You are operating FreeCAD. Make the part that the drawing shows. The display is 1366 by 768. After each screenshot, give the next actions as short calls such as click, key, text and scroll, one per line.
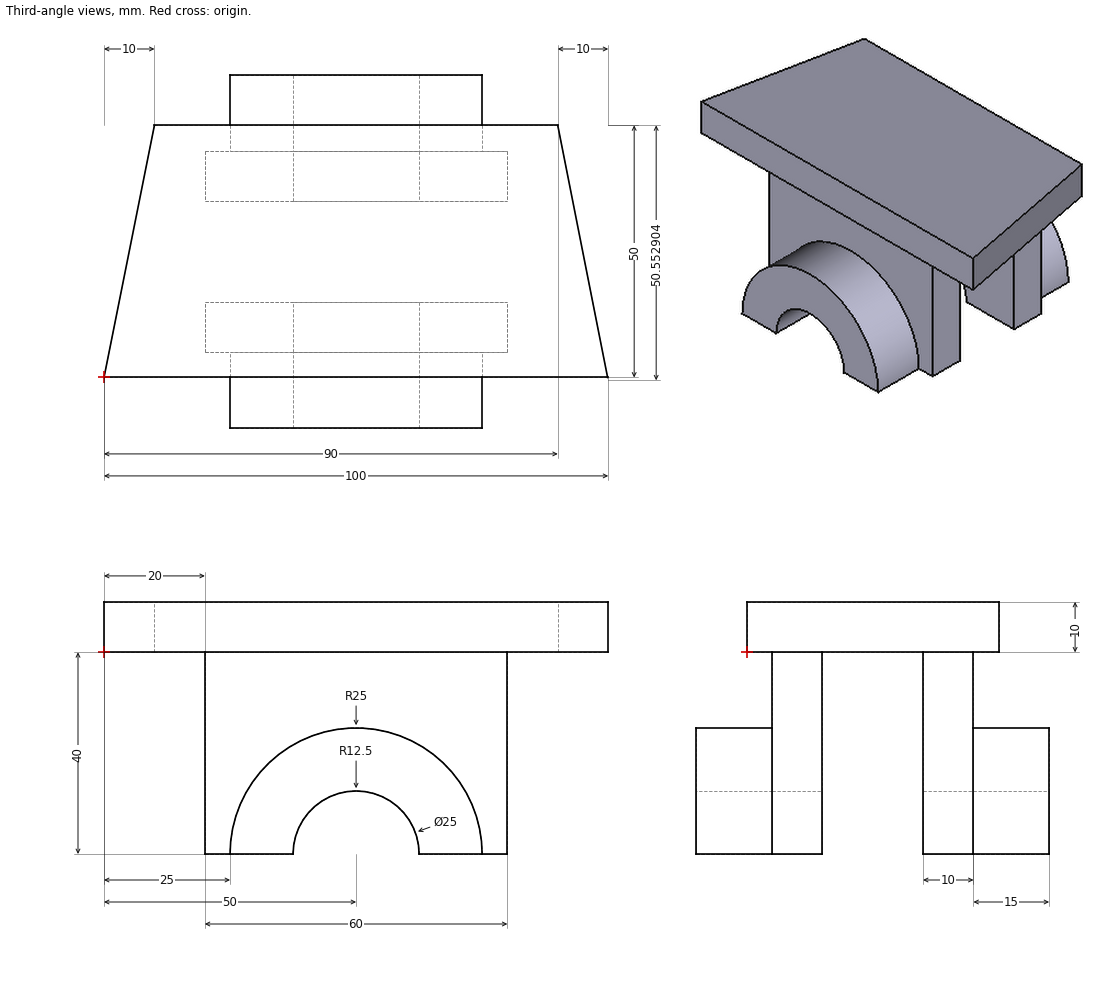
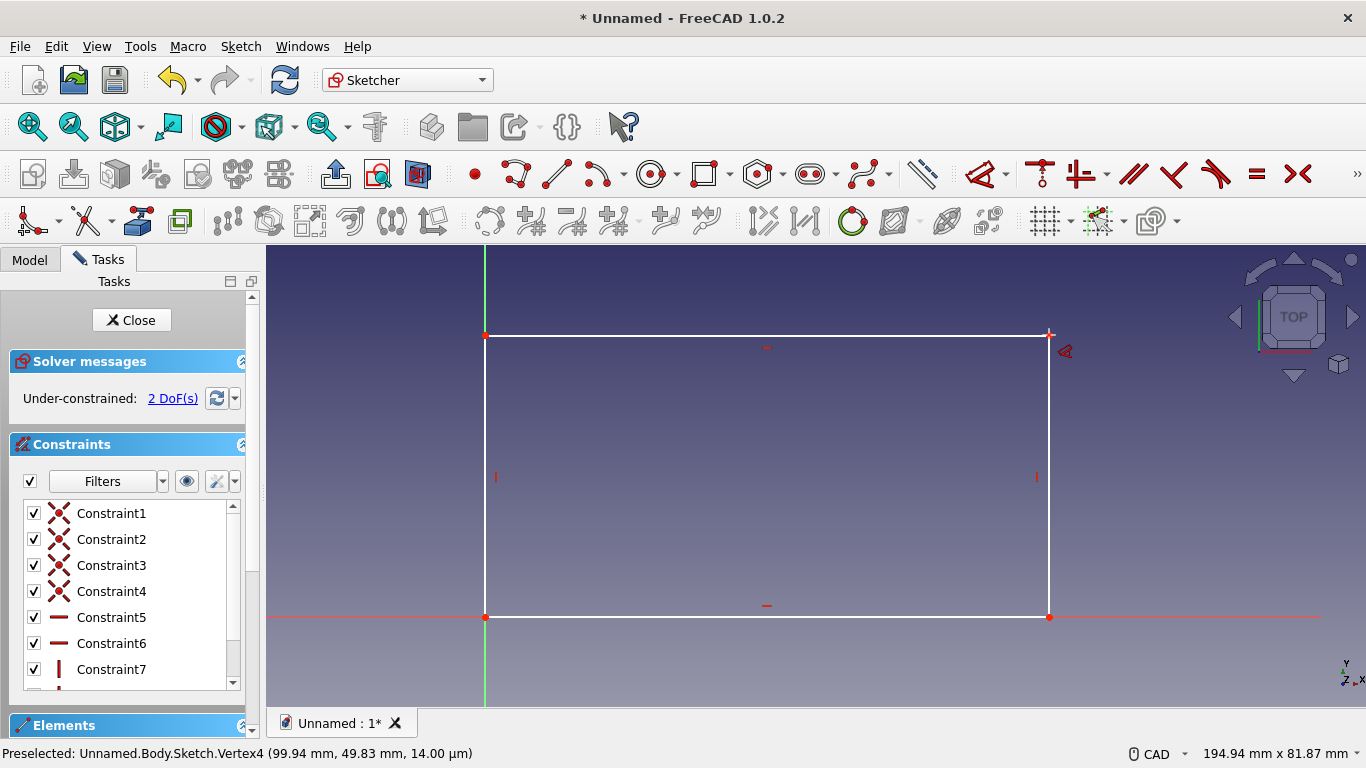
click(1049, 533)
click(1083, 477)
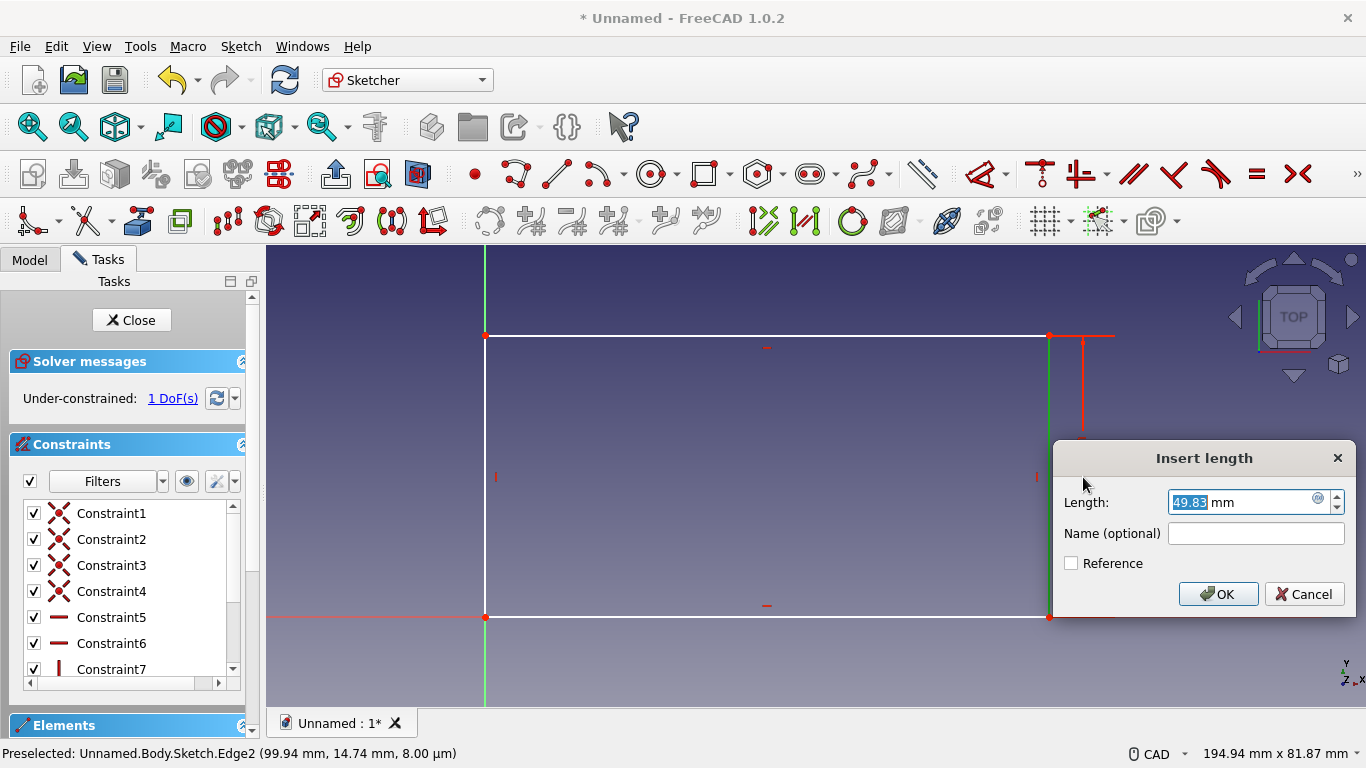
text(50)
key(Return)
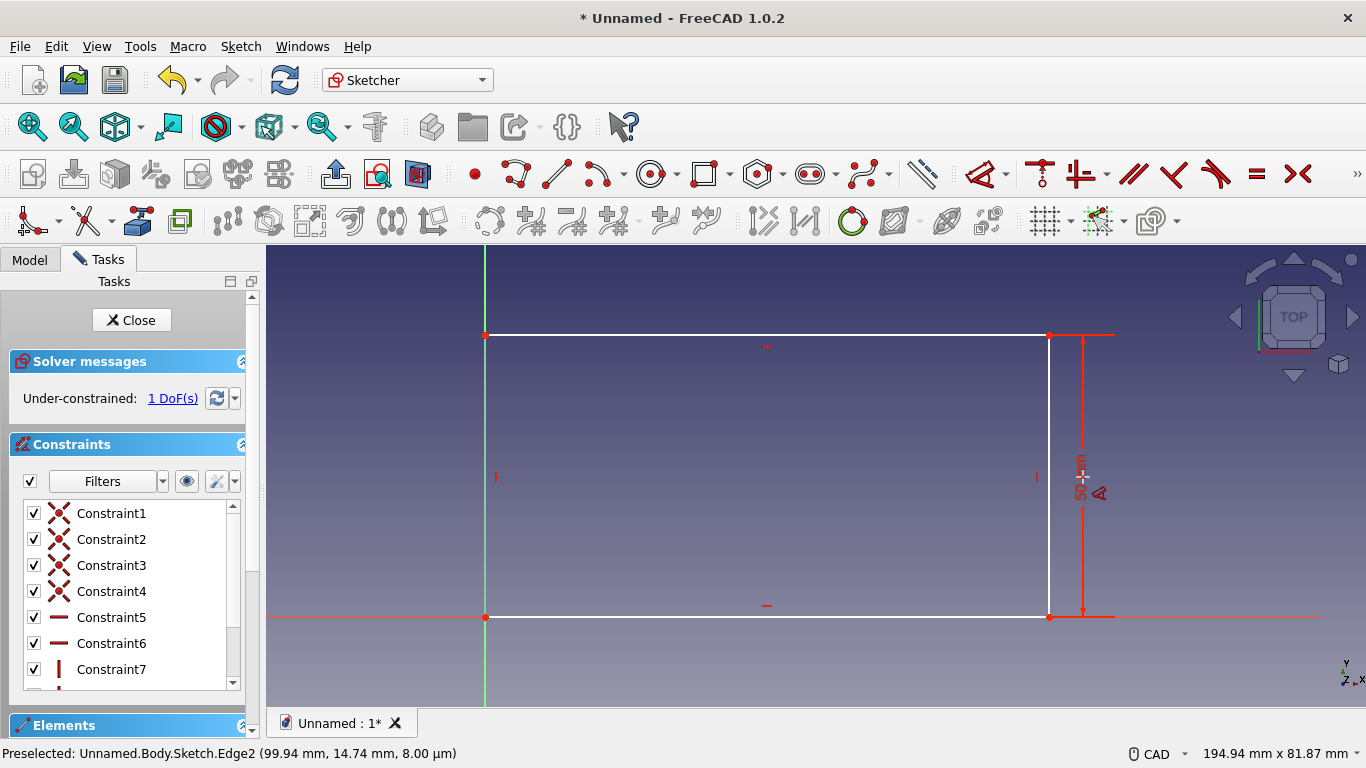
click(654, 617)
click(767, 651)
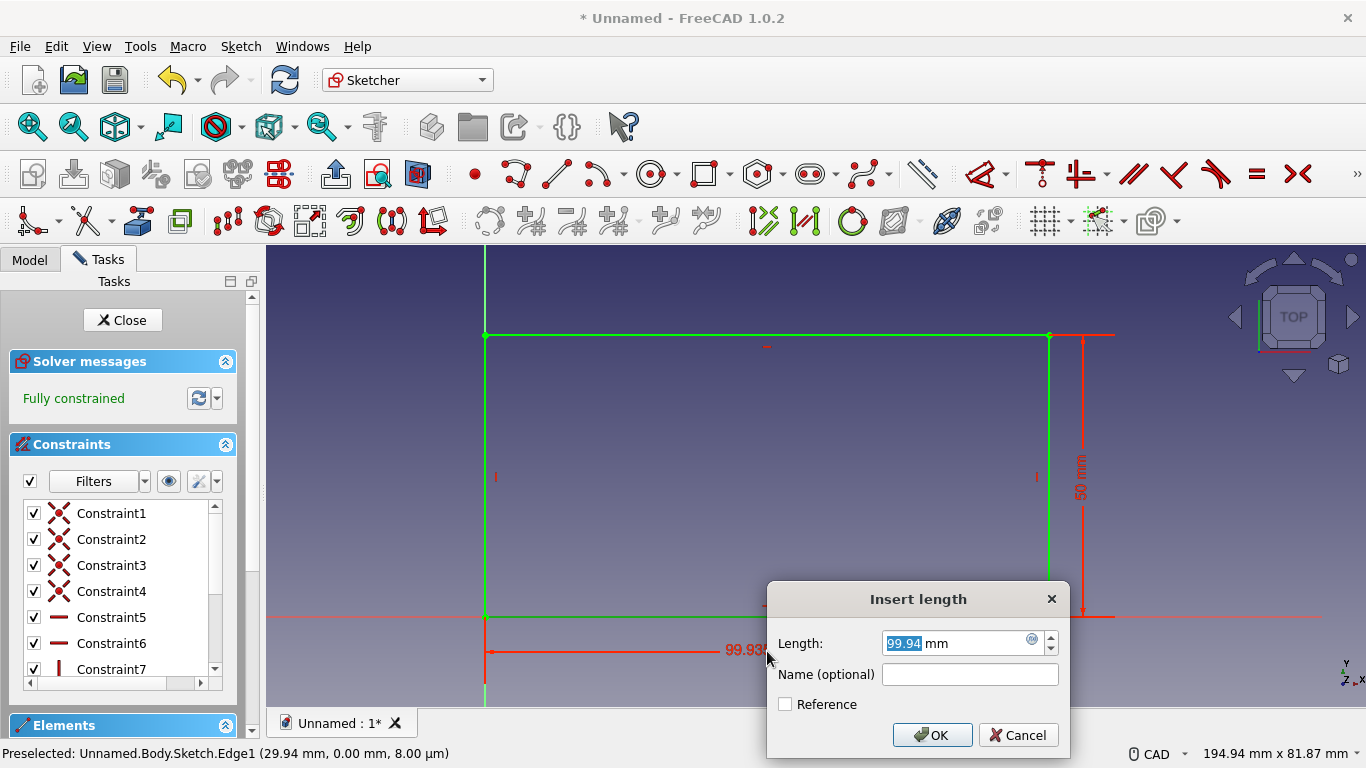
text(100)
key(Return)
key(Escape)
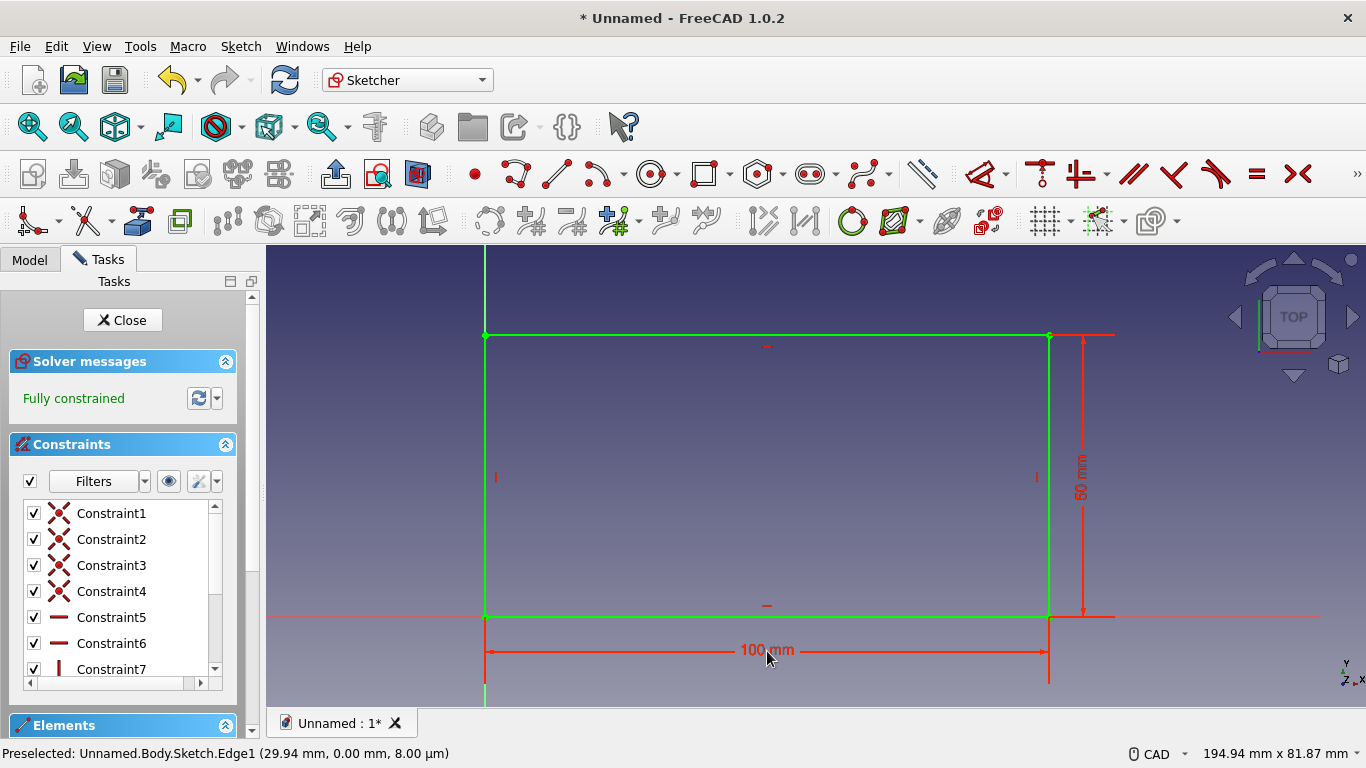
click(123, 320)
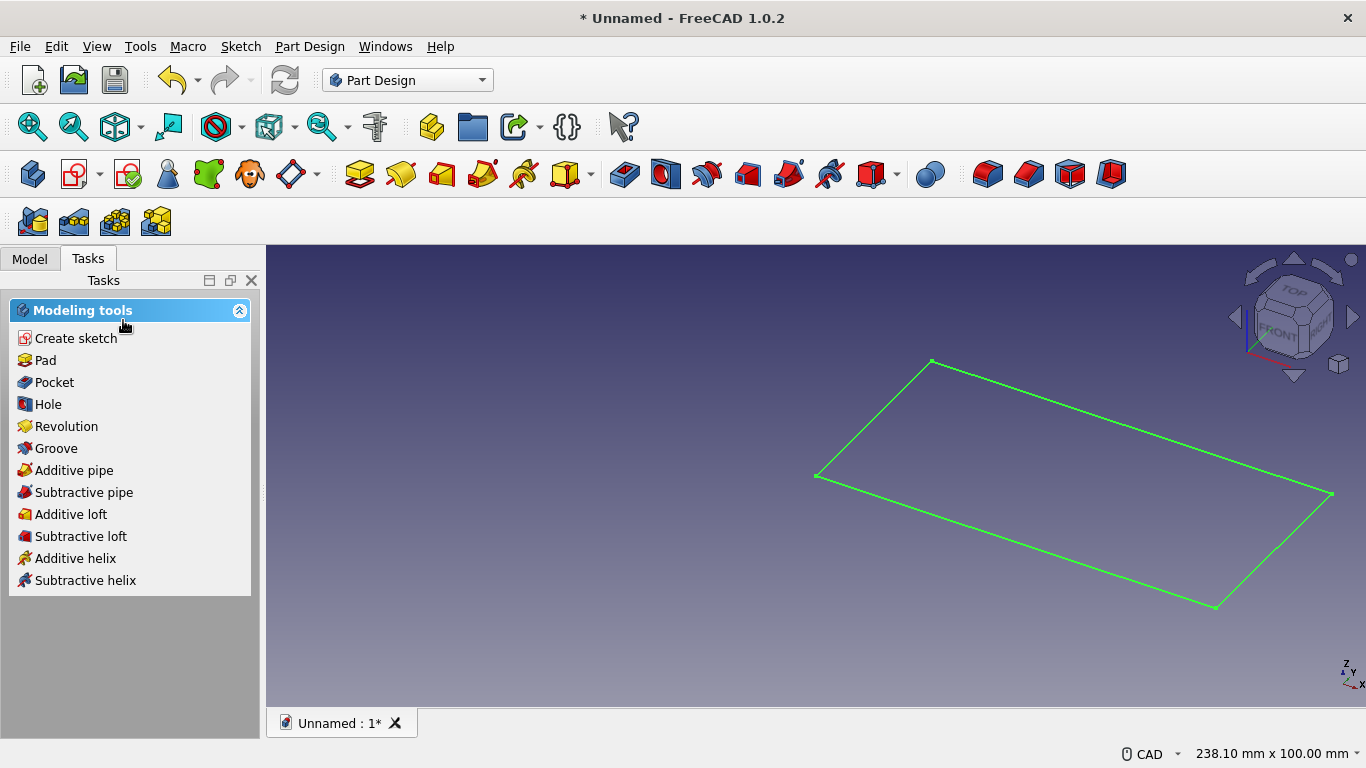
click(360, 174)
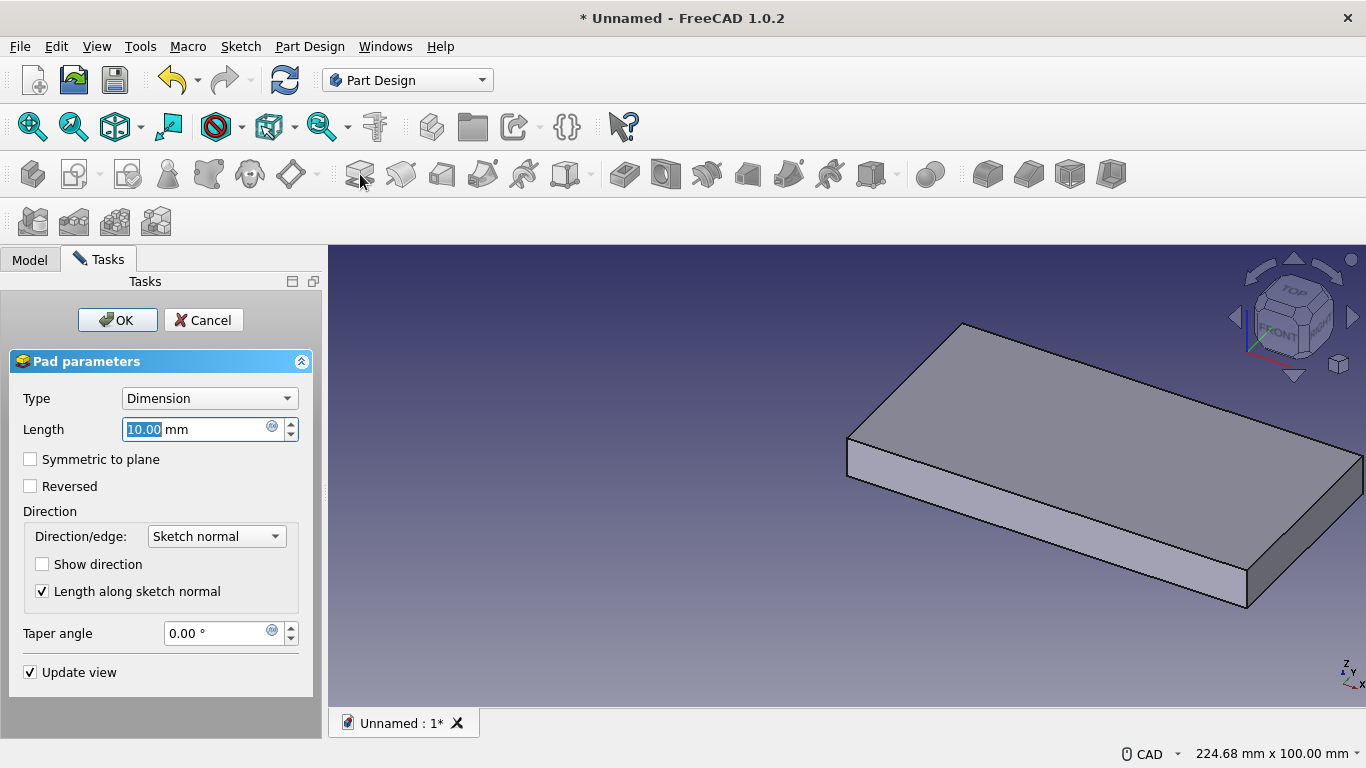
text(10)
key(Tab)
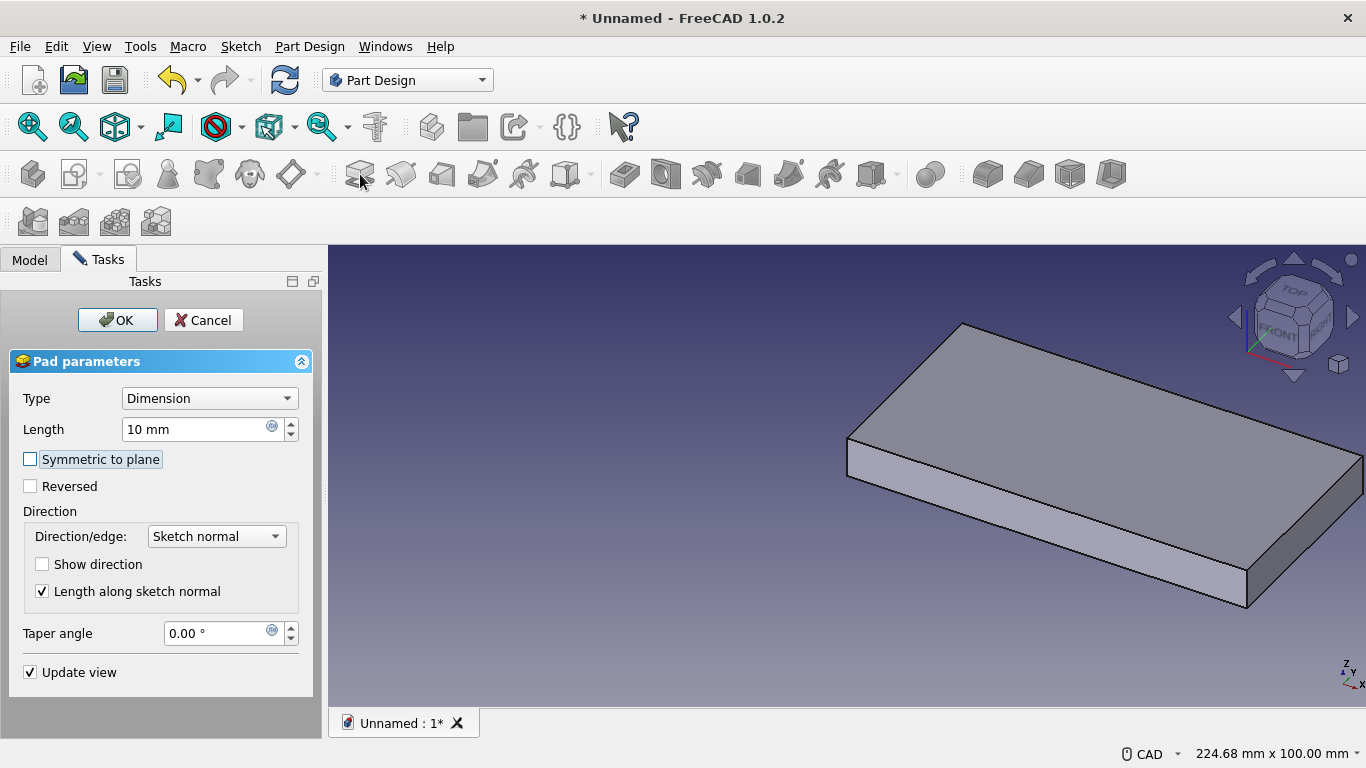
click(118, 320)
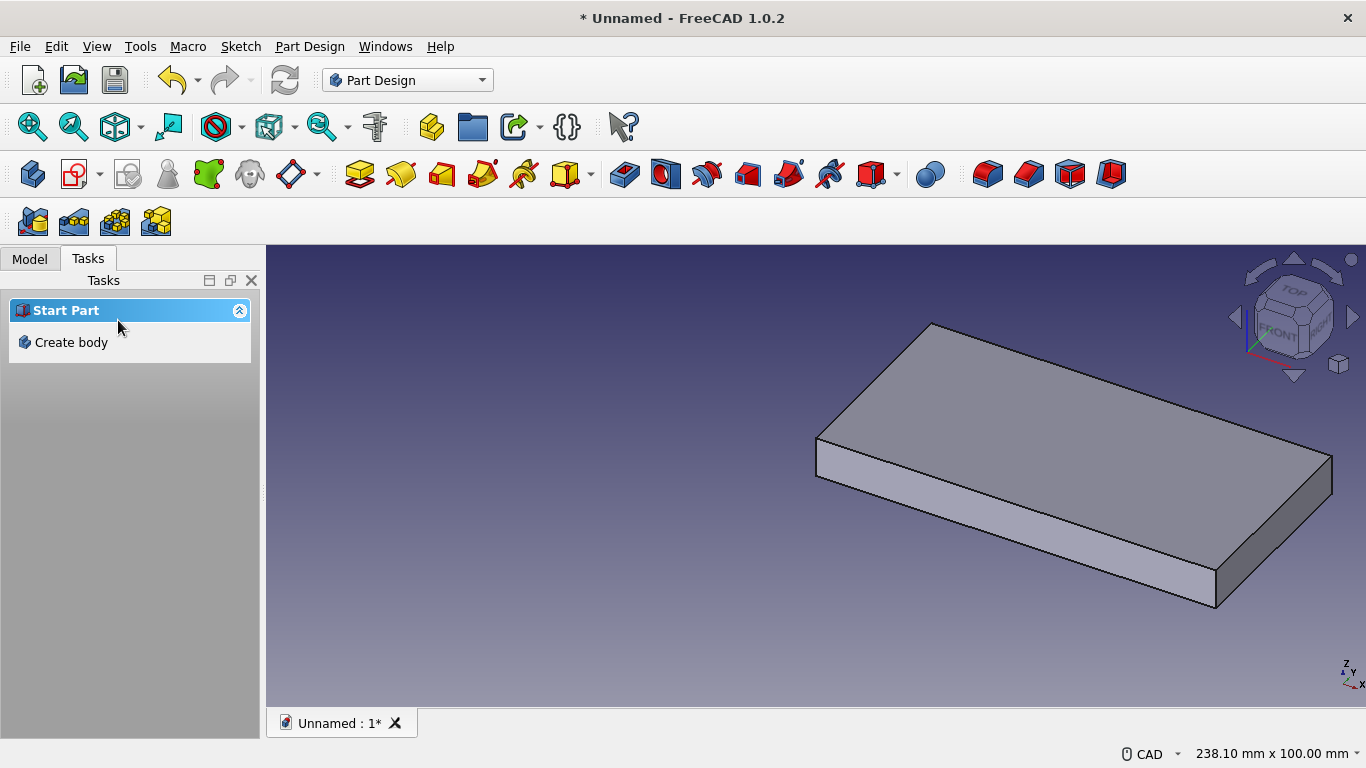
click(30, 258)